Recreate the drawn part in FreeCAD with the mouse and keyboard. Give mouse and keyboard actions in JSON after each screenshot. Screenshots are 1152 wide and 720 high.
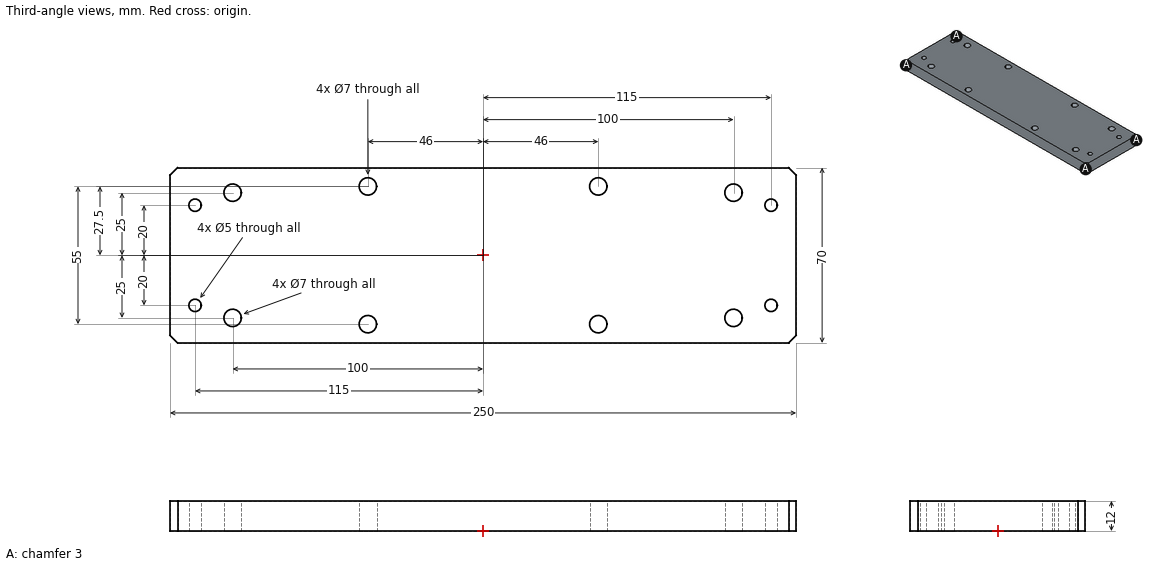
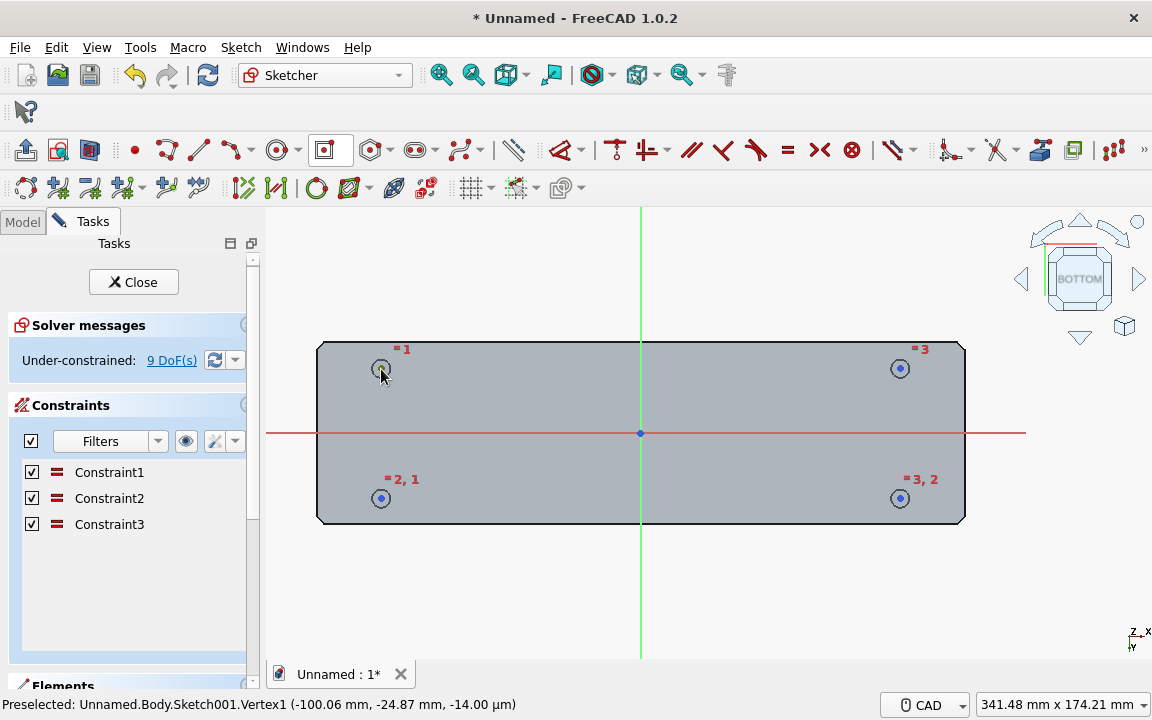
{"action": "left_click", "coordinate": [381, 499]}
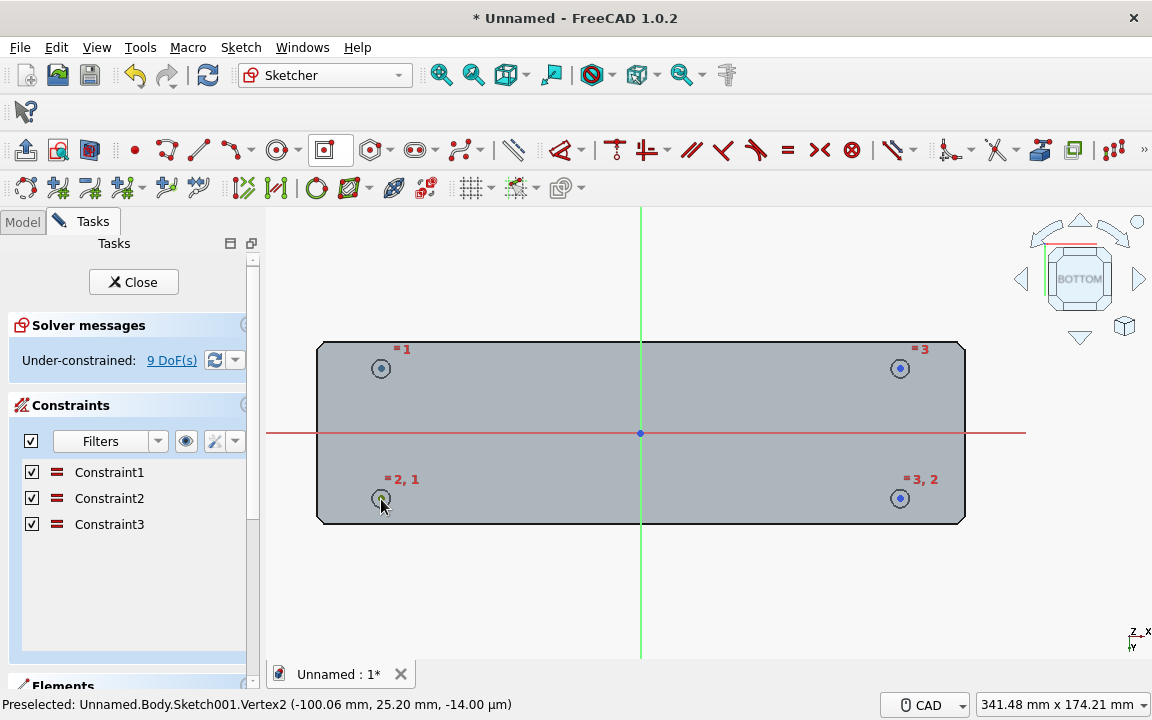
{"action": "left_click", "coordinate": [670, 150]}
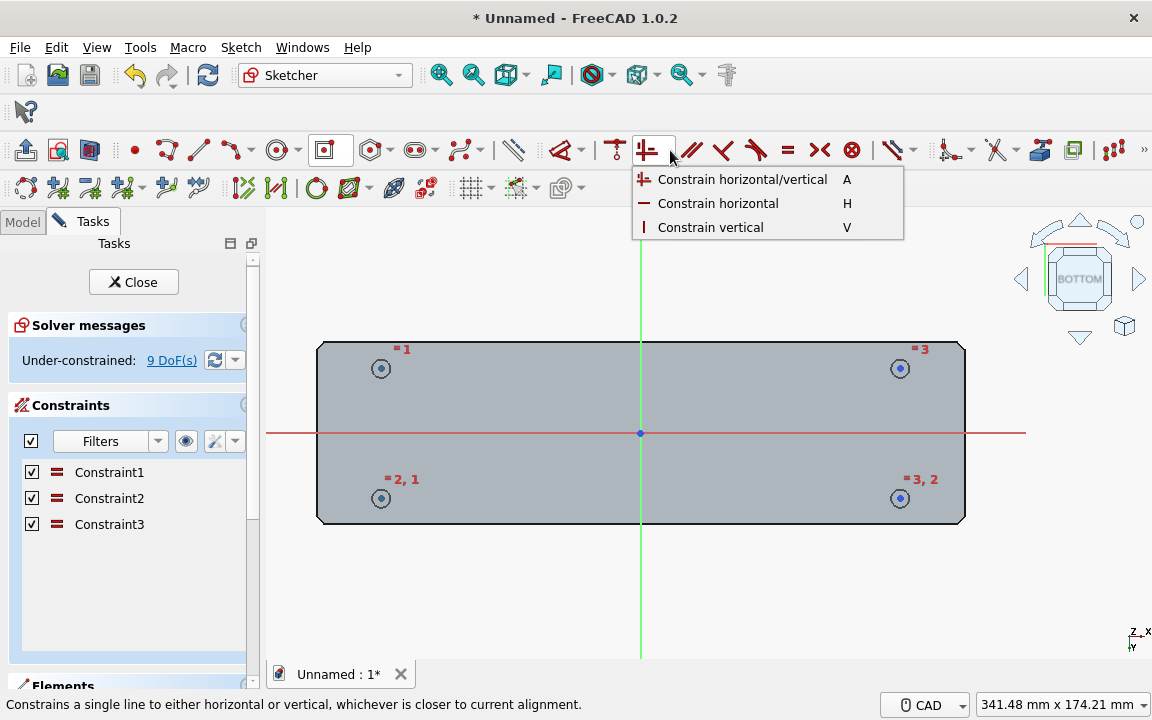
{"action": "left_click", "coordinate": [768, 227]}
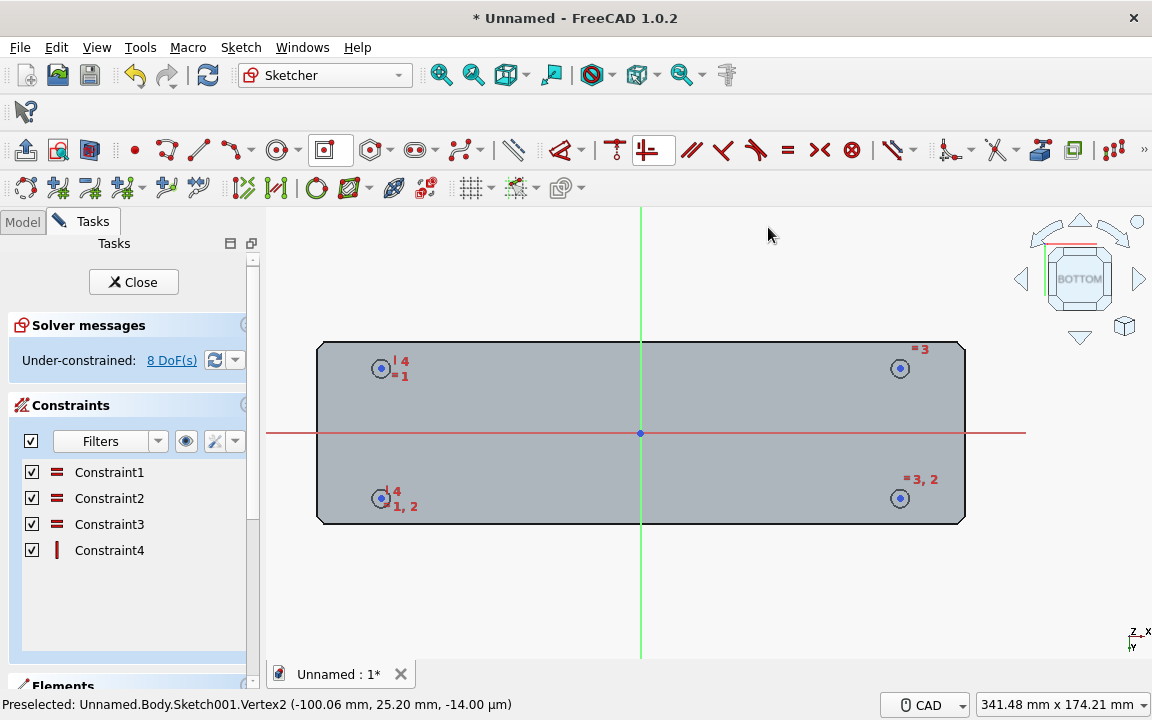
{"action": "left_click", "coordinate": [381, 499]}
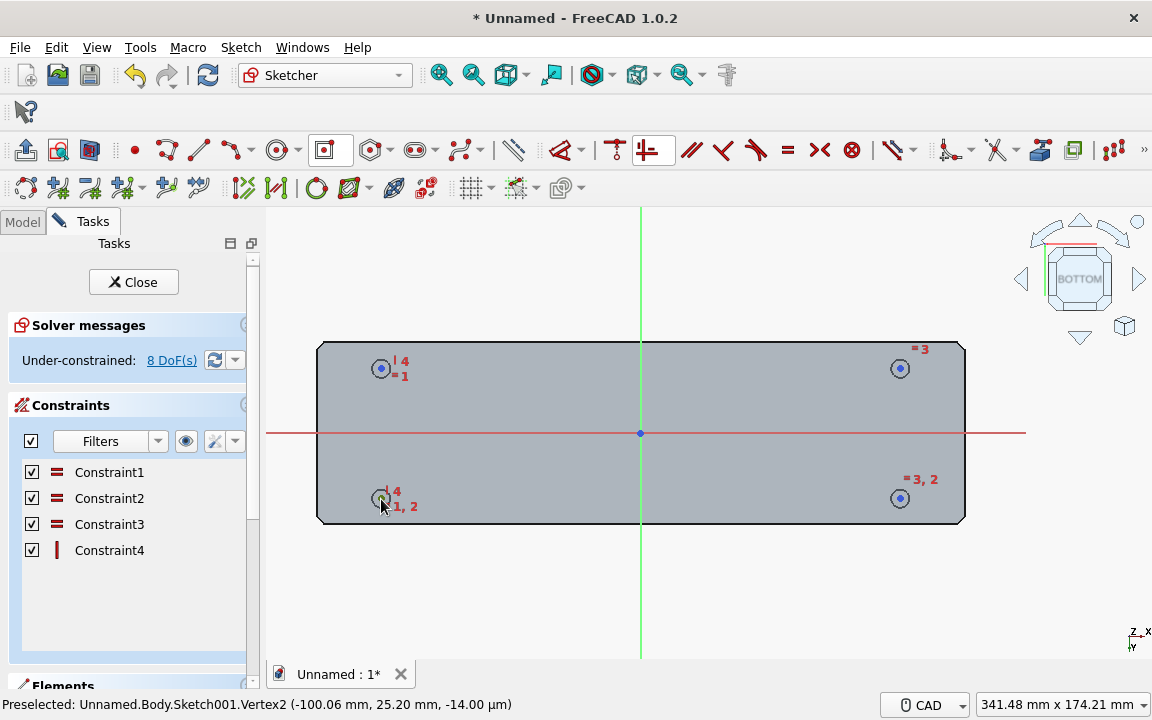
{"action": "left_click", "coordinate": [900, 499]}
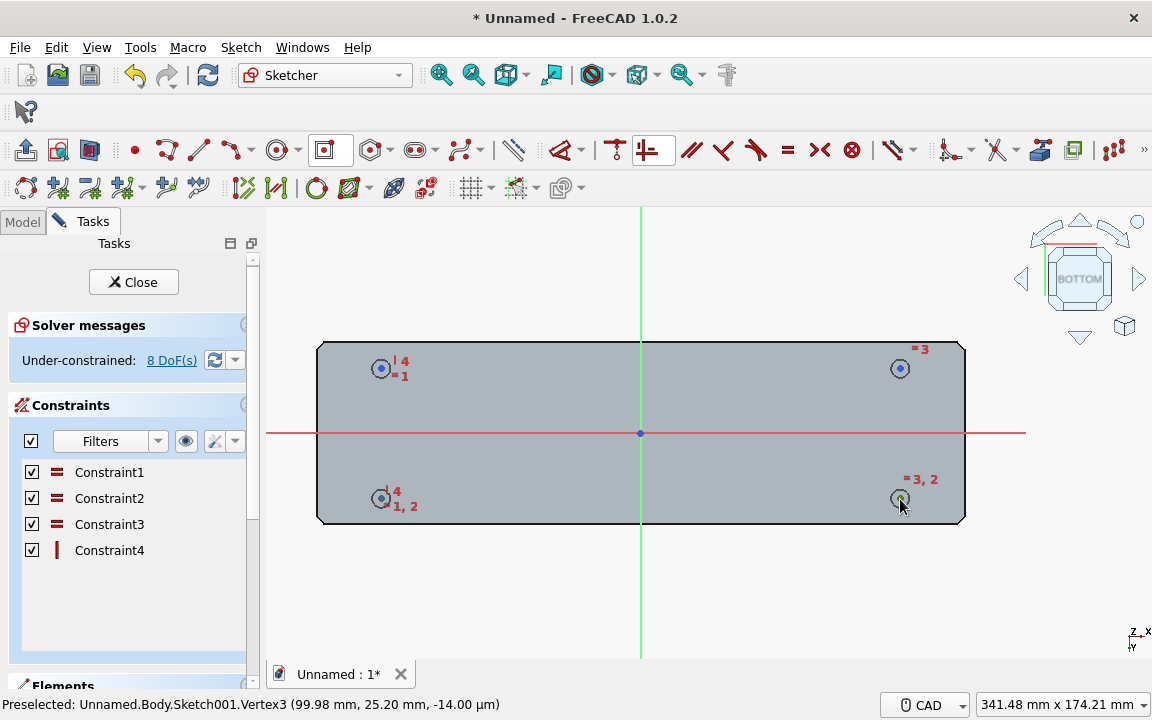
{"action": "left_click", "coordinate": [670, 150]}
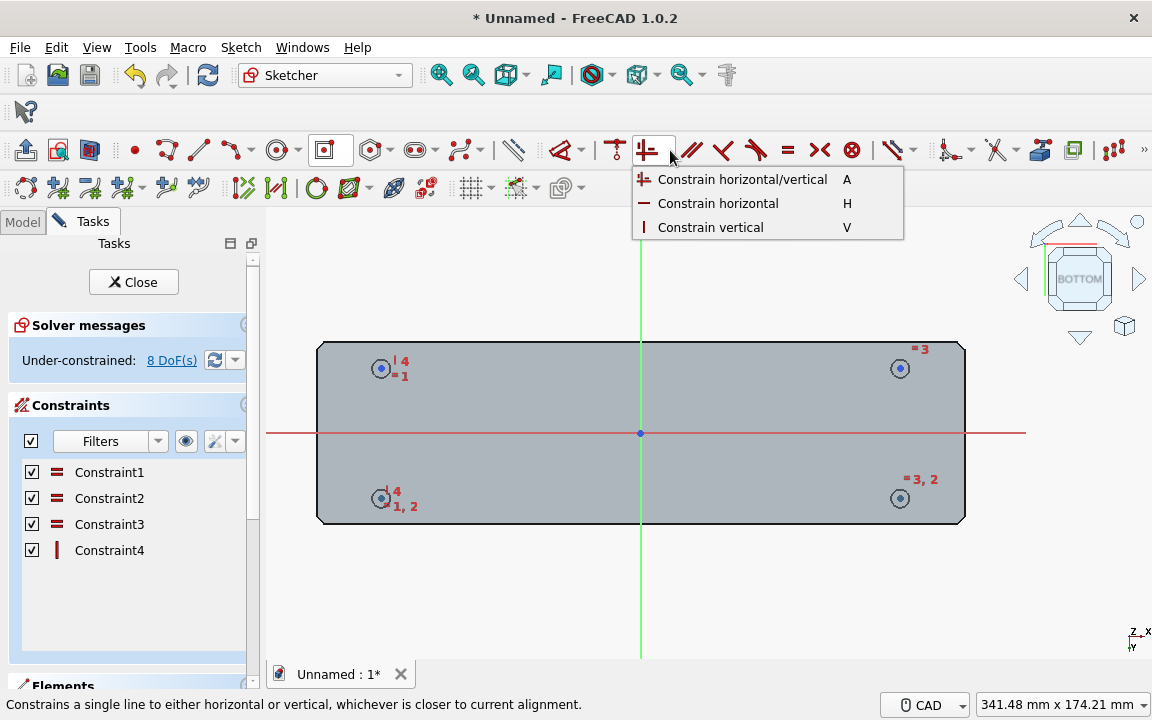
{"action": "left_click", "coordinate": [768, 203]}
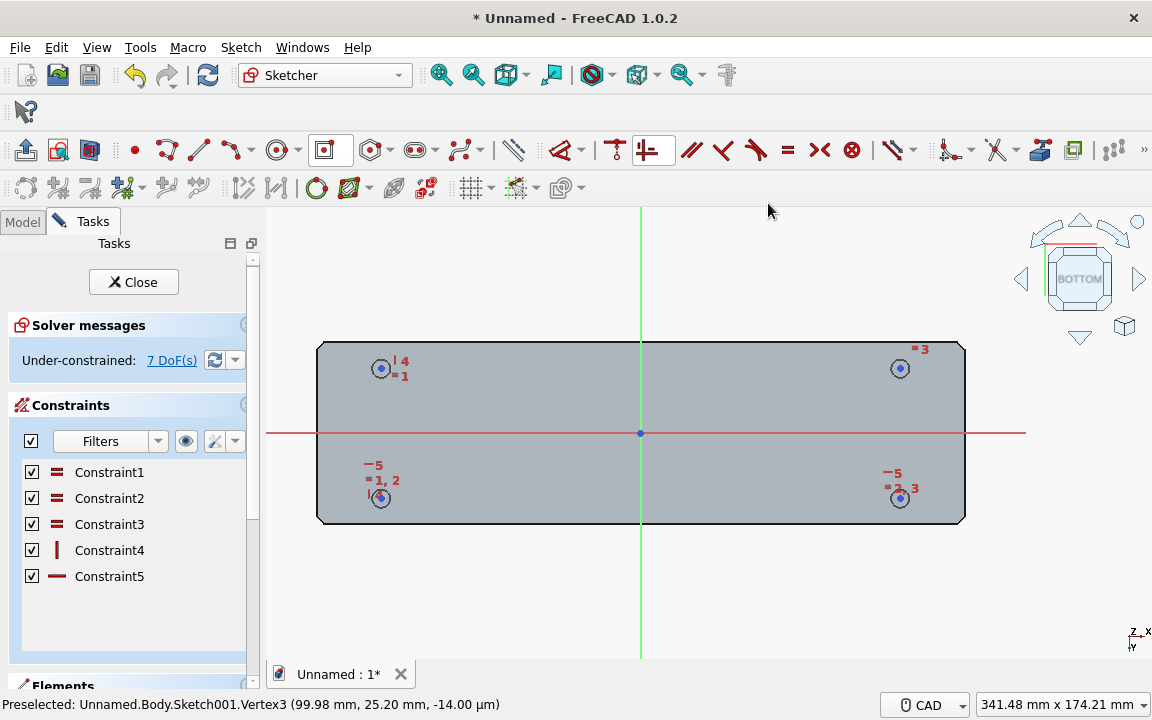
{"action": "left_click", "coordinate": [900, 499]}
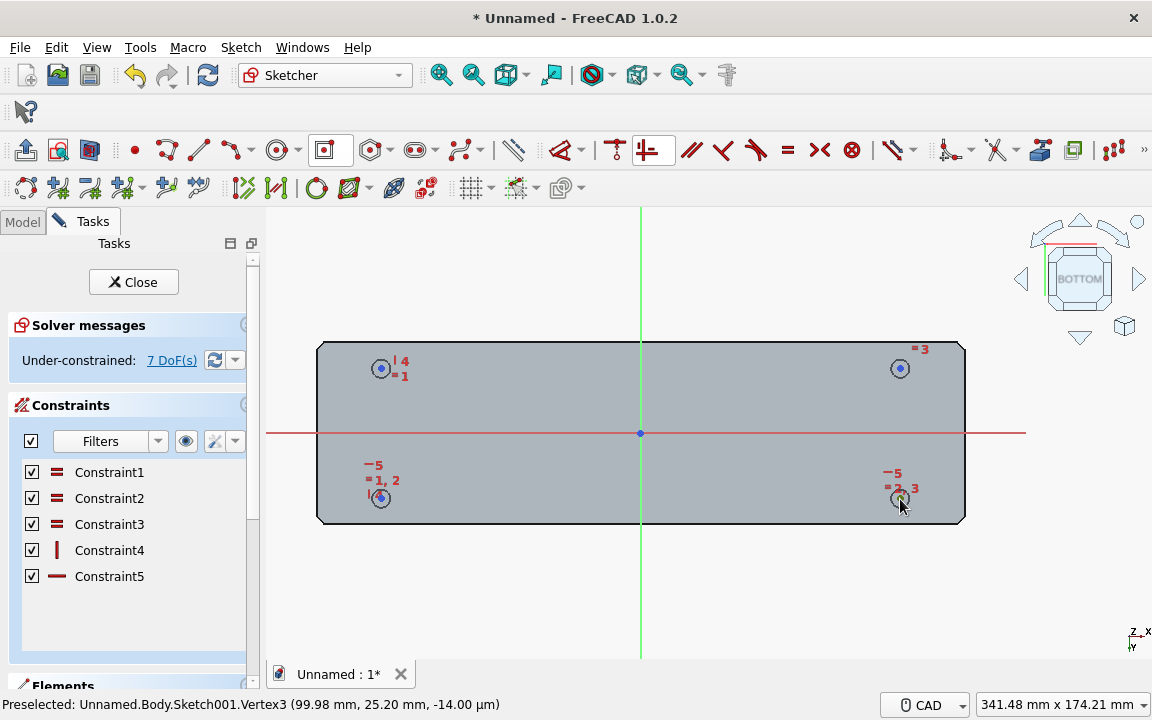
{"action": "left_click", "coordinate": [900, 369]}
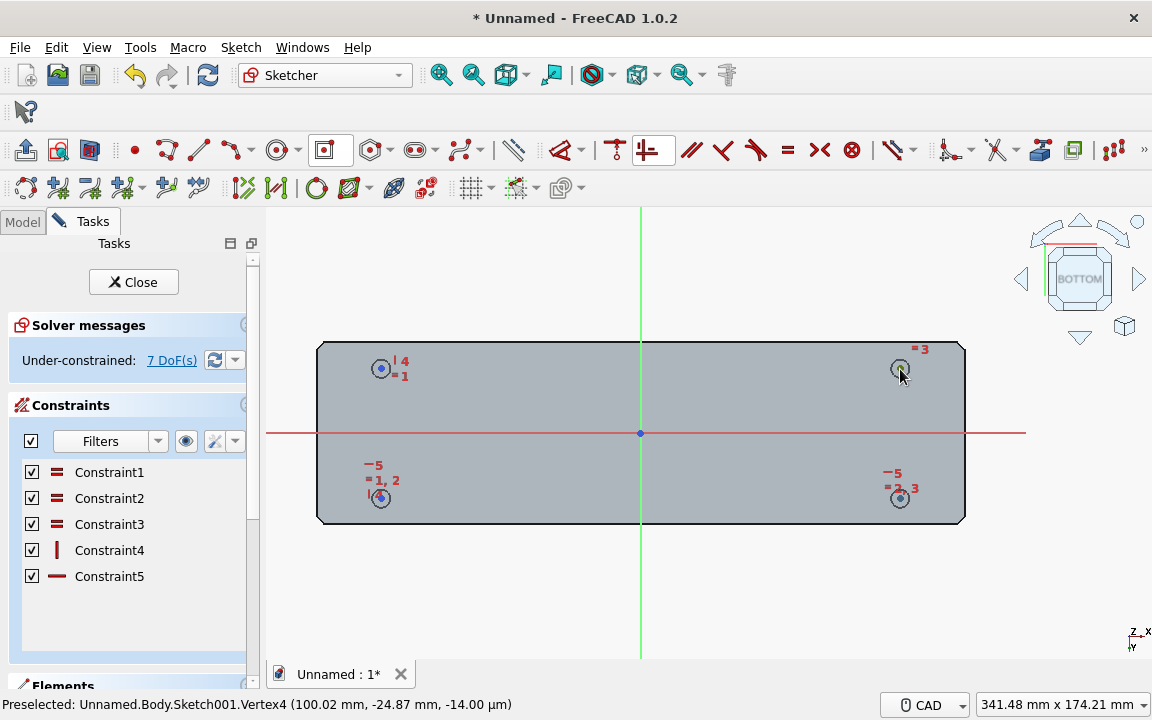
{"action": "key", "text": "v"}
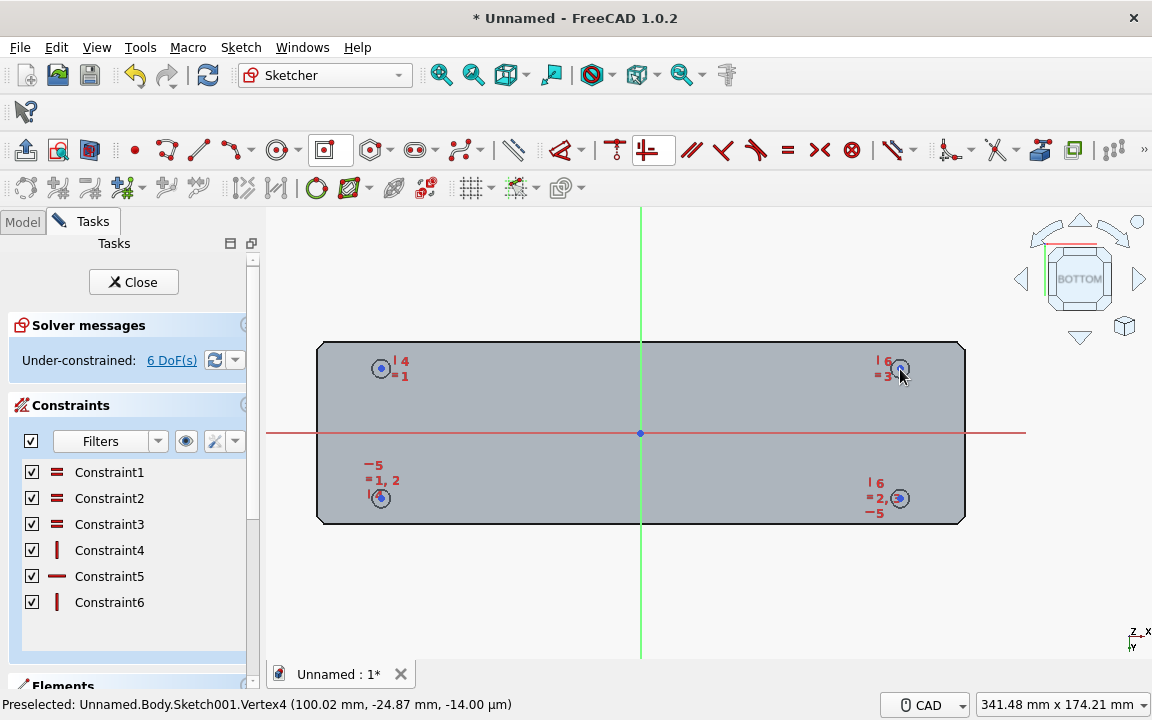
{"action": "left_click", "coordinate": [381, 369]}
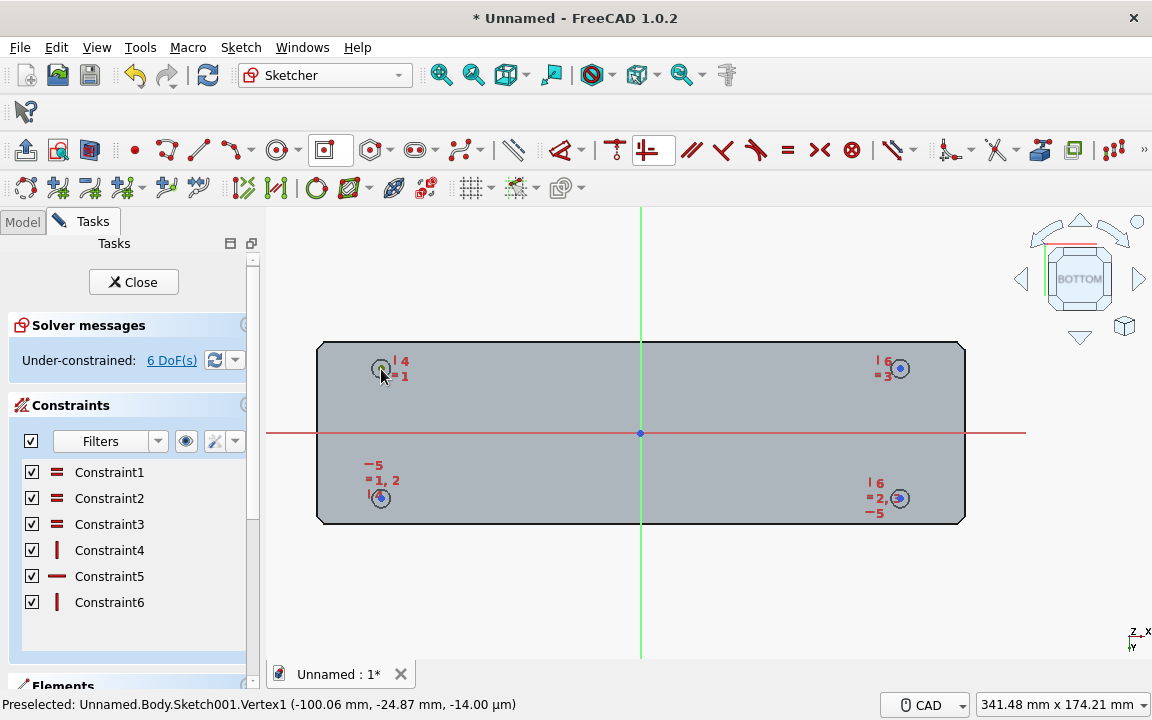
{"action": "left_click", "coordinate": [900, 369]}